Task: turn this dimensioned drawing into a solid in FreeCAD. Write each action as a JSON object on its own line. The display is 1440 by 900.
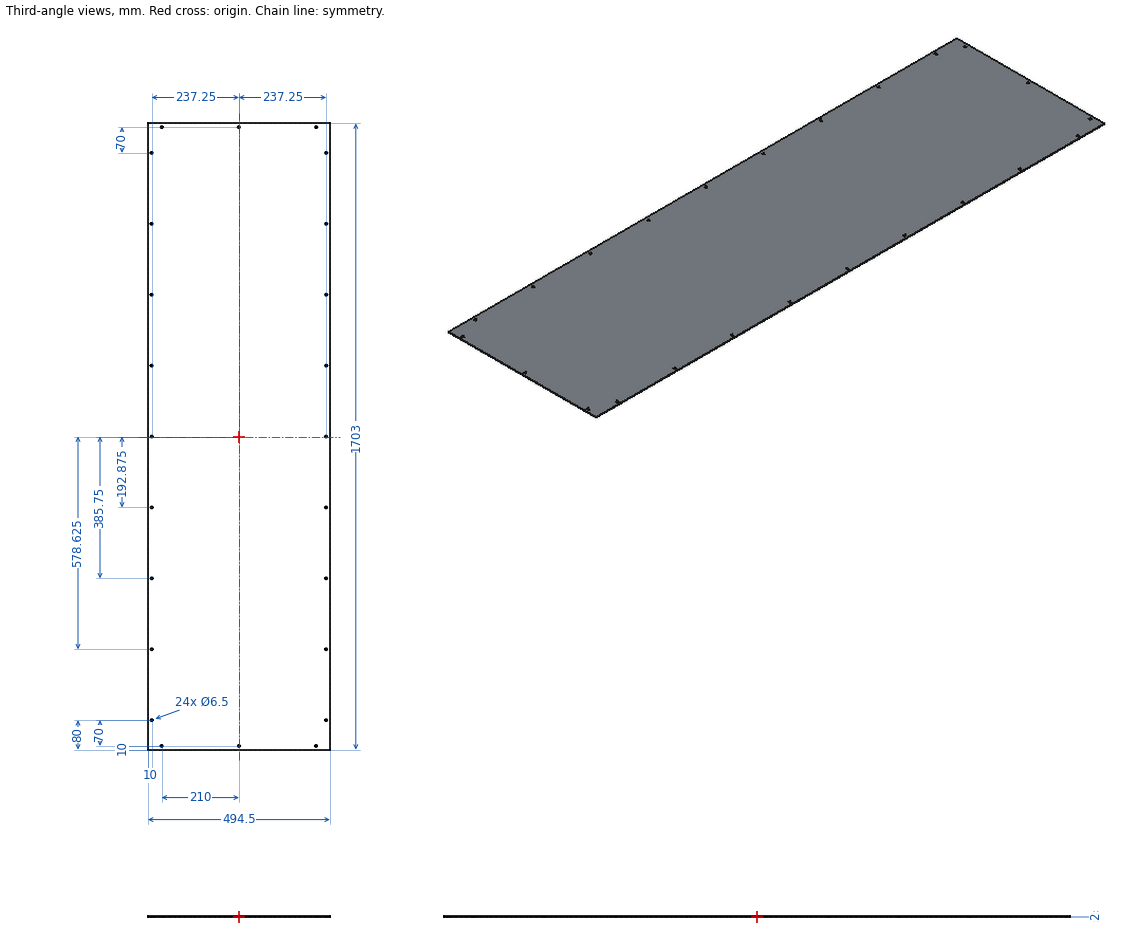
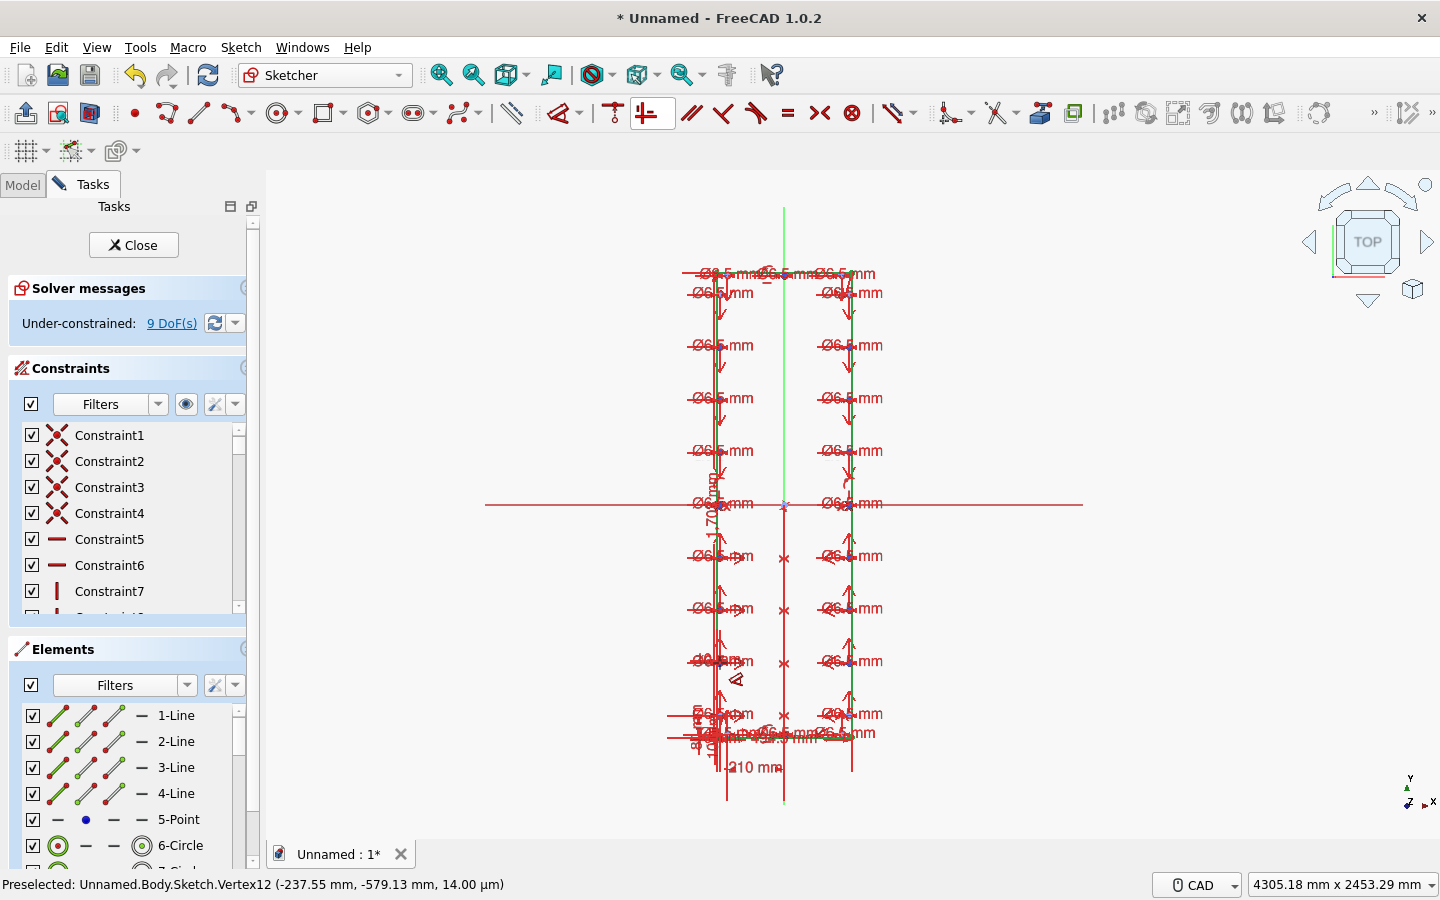
{"action": "scroll", "coordinate": [717, 738], "scroll_direction": "up", "scroll_amount": 14}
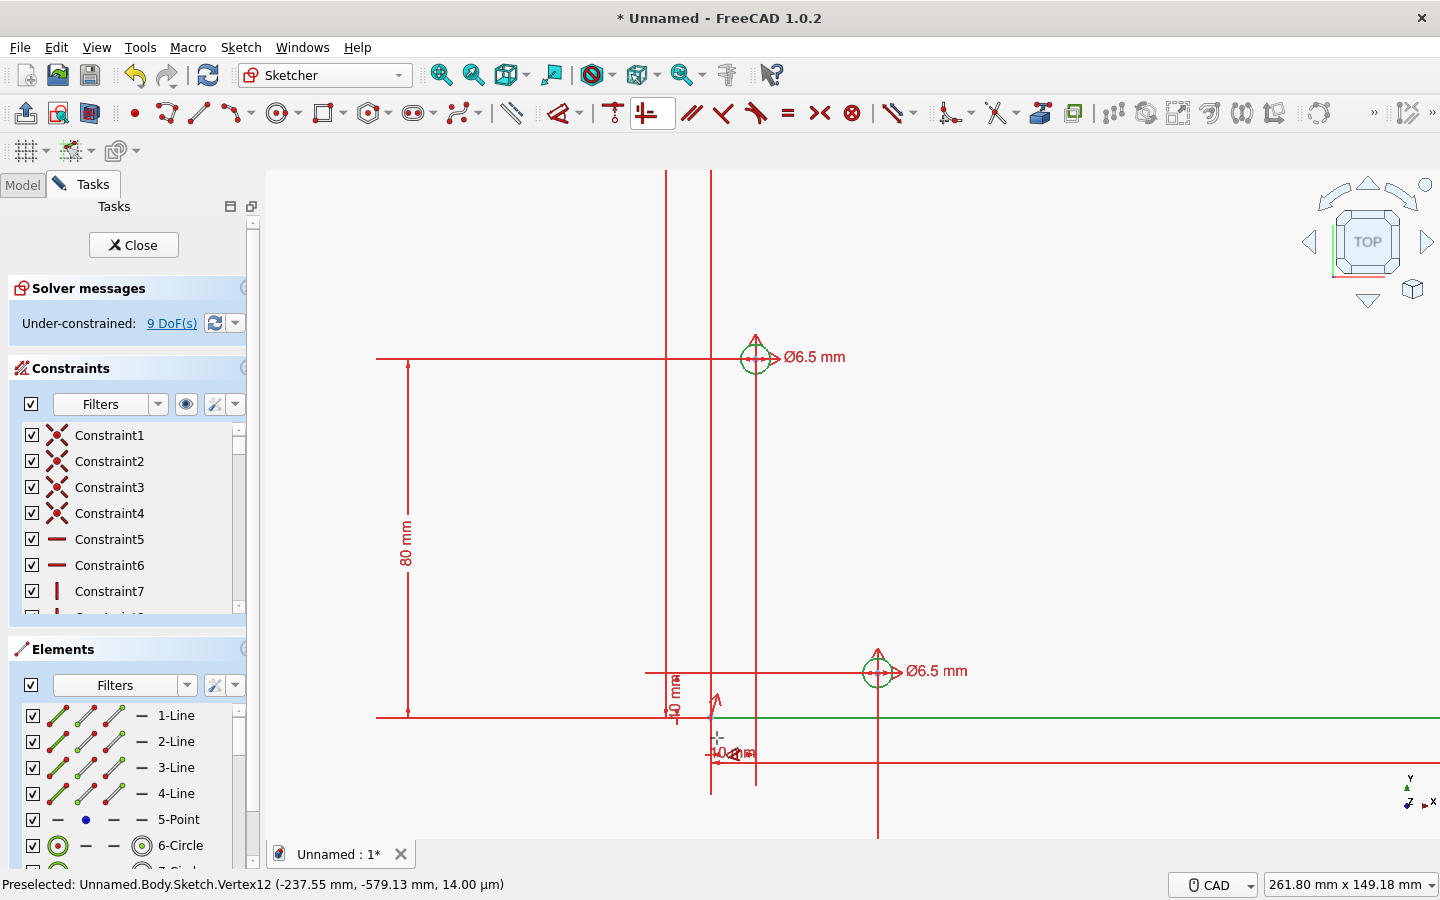
{"action": "left_click", "coordinate": [711, 718]}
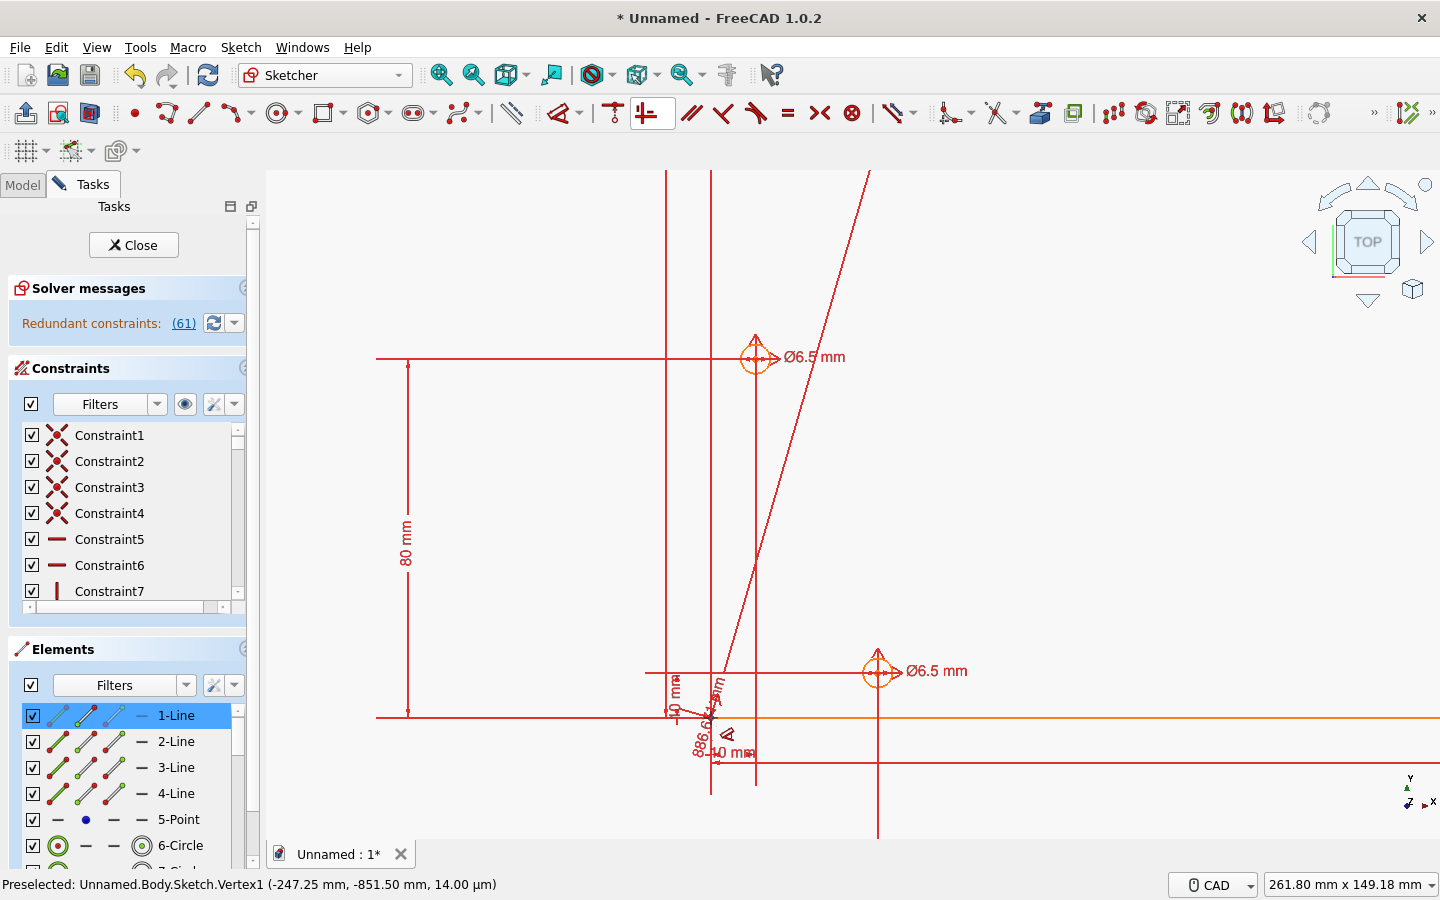
{"action": "scroll", "coordinate": [717, 738], "scroll_direction": "down", "scroll_amount": 14}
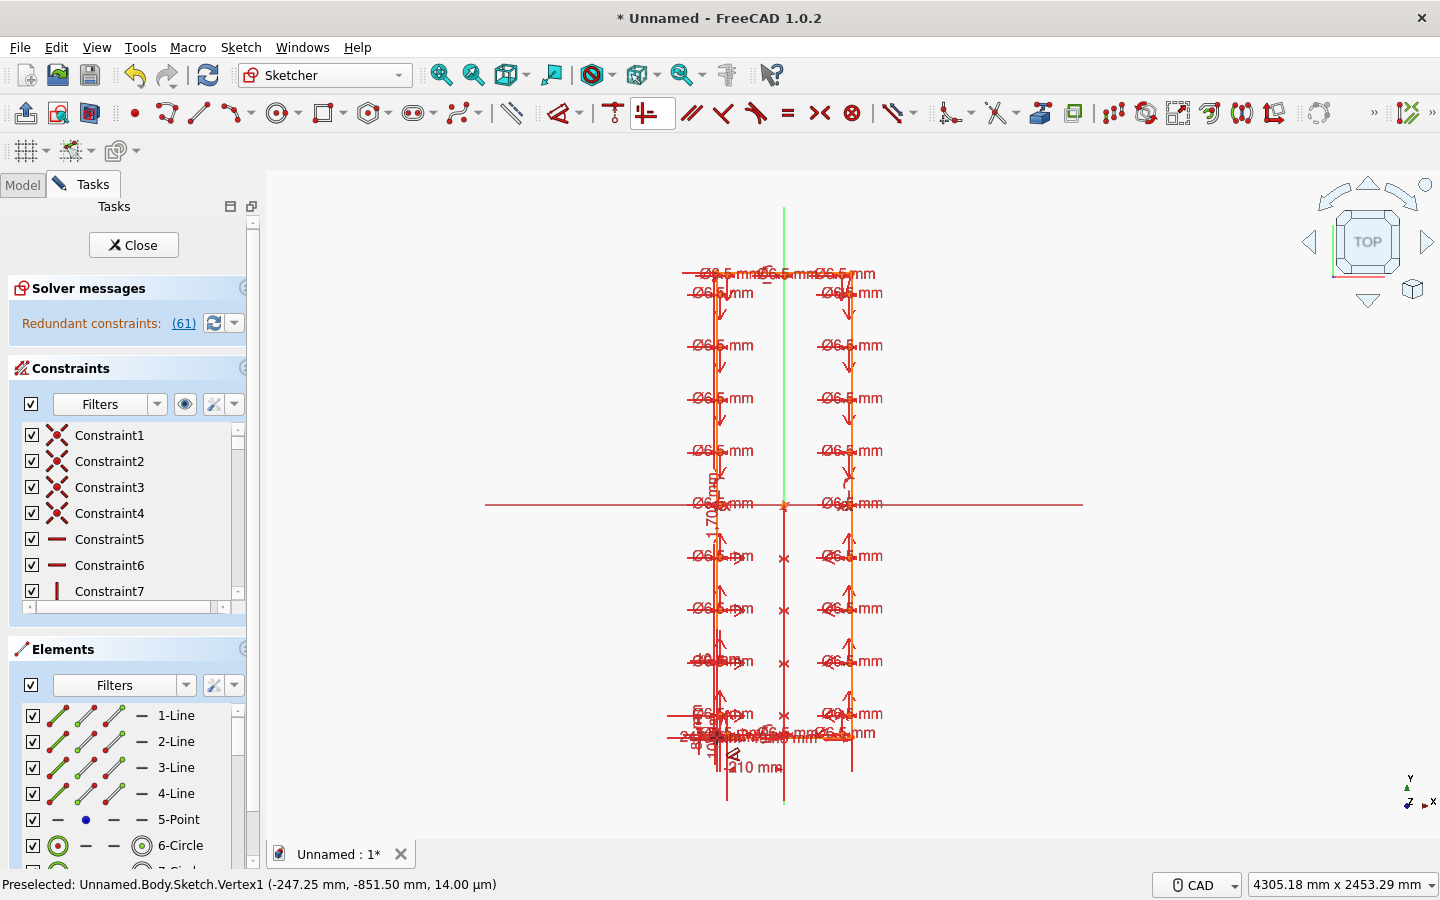
{"action": "scroll", "coordinate": [720, 610], "scroll_direction": "up", "scroll_amount": 14}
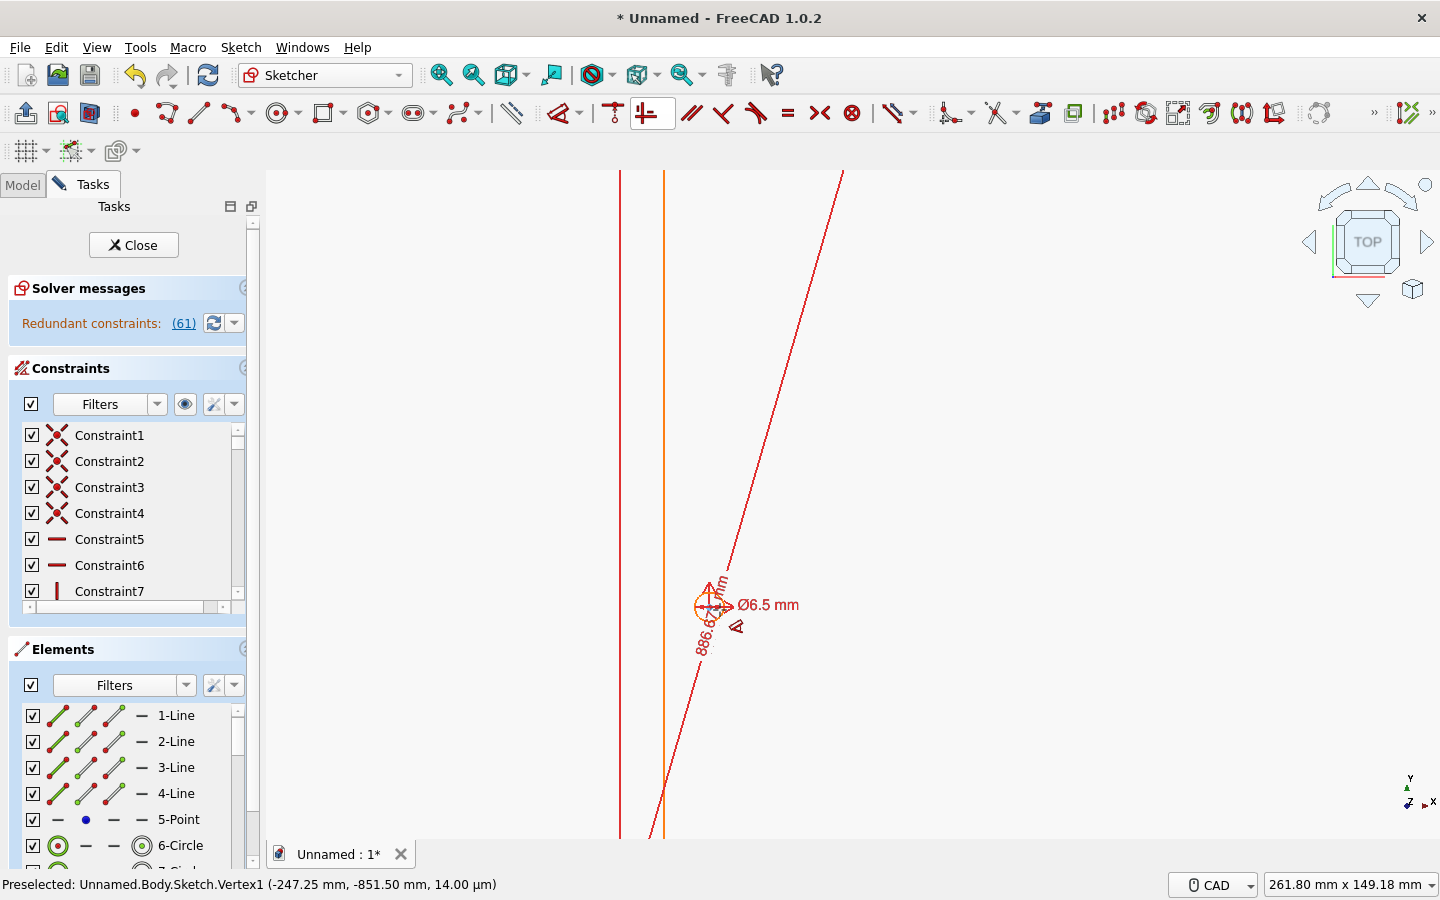
{"action": "left_click", "coordinate": [709, 607]}
{"action": "left_click", "coordinate": [687, 573]}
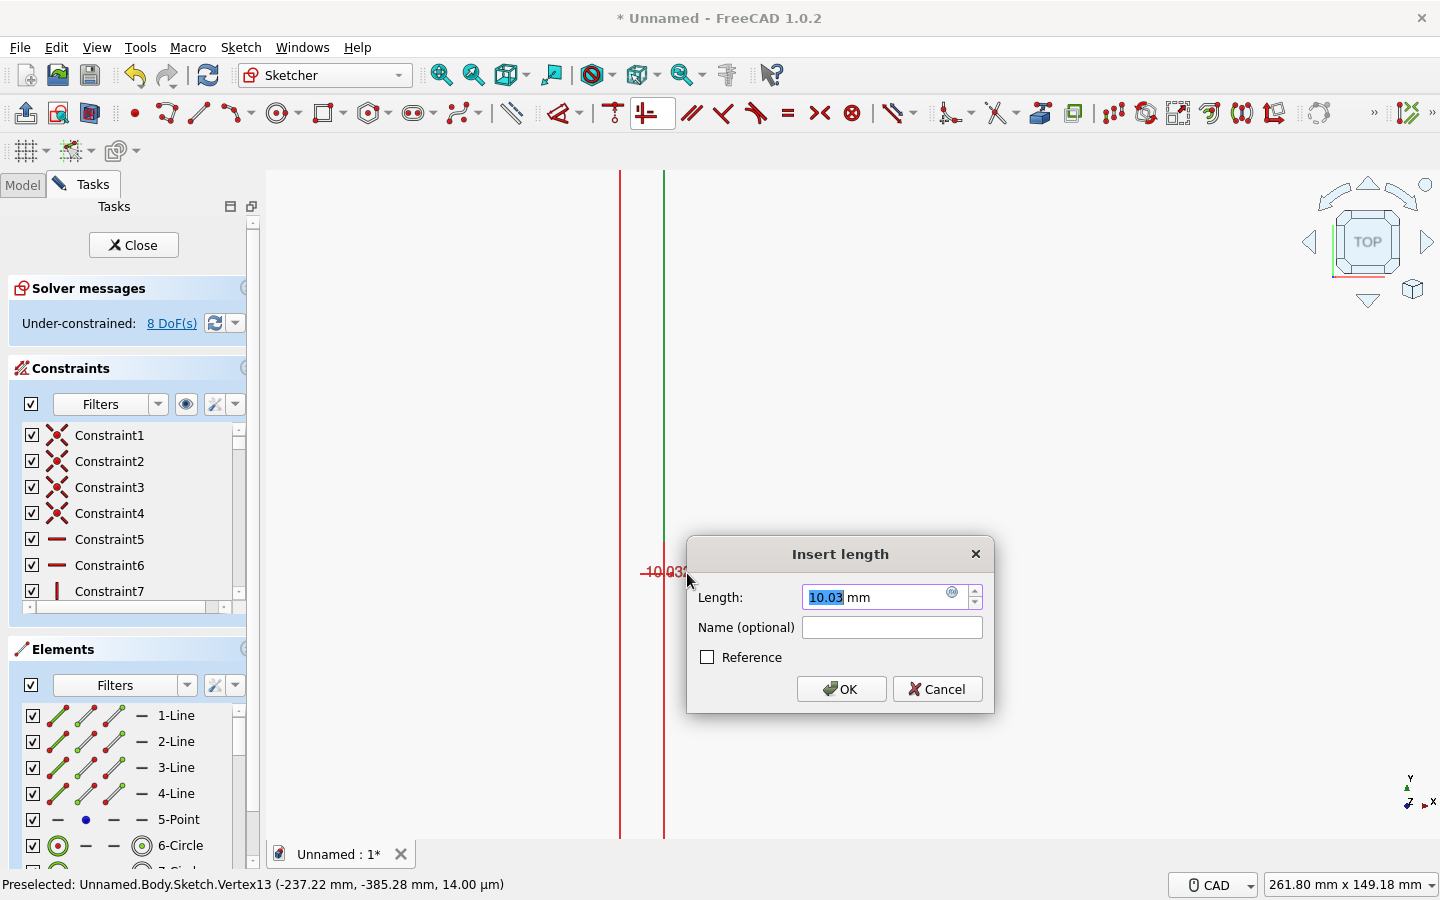
{"action": "type", "text": "10"}
{"action": "key", "text": "Return"}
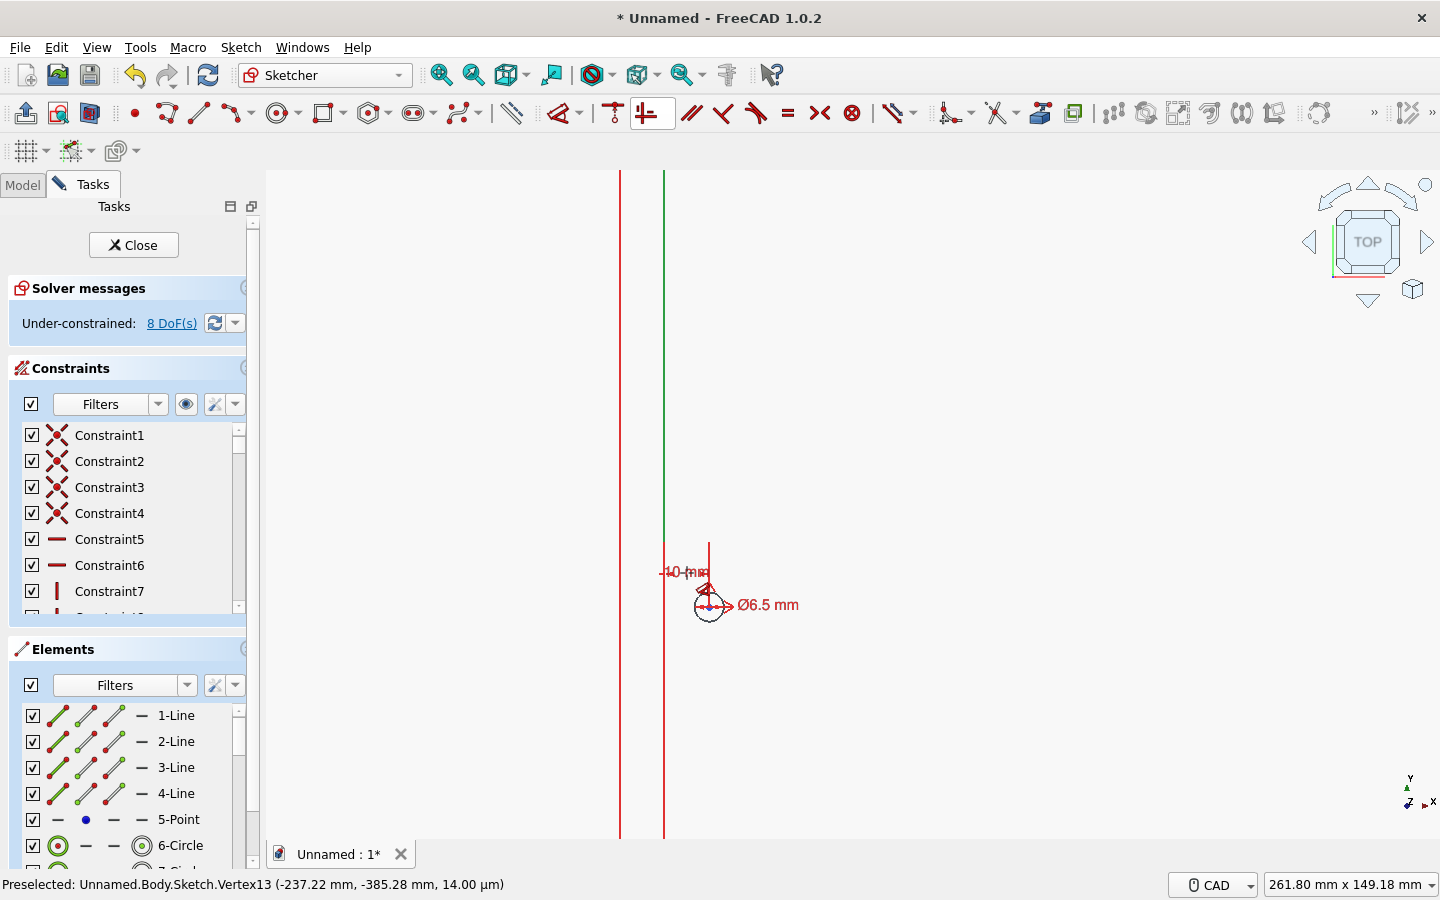
{"action": "scroll", "coordinate": [720, 610], "scroll_direction": "down", "scroll_amount": 14}